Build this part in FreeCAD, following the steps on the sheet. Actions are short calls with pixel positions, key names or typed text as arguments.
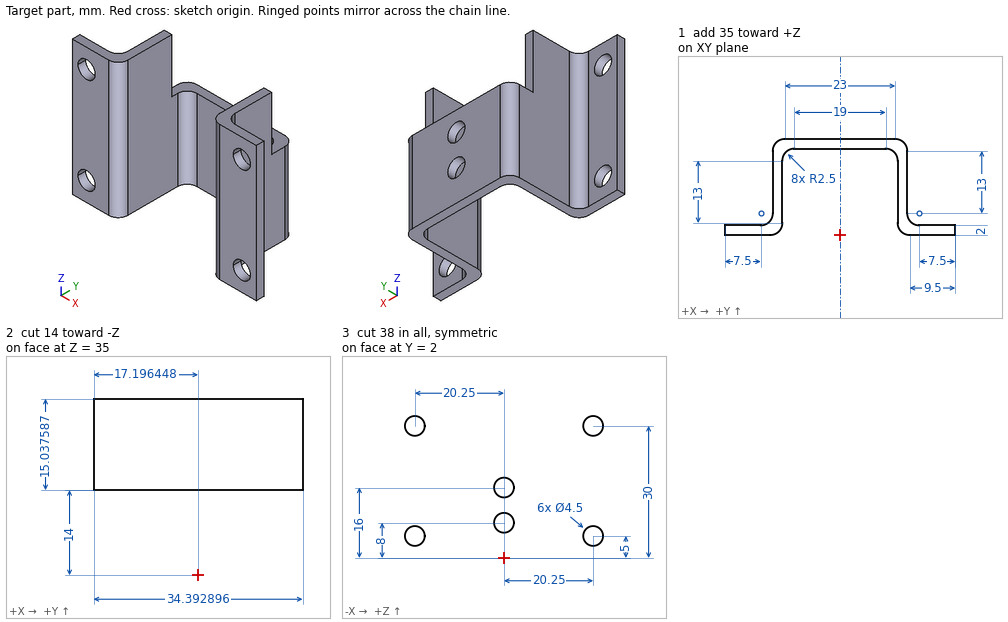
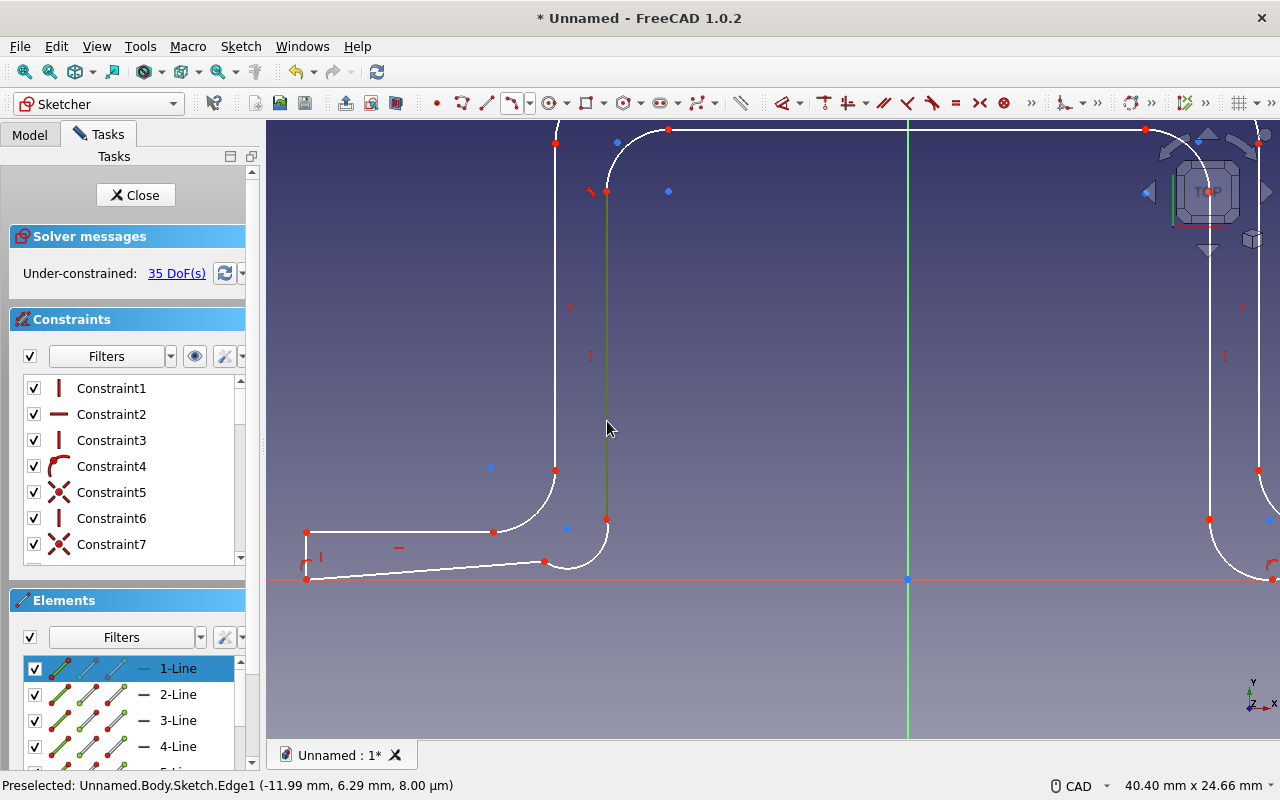
click(572, 568)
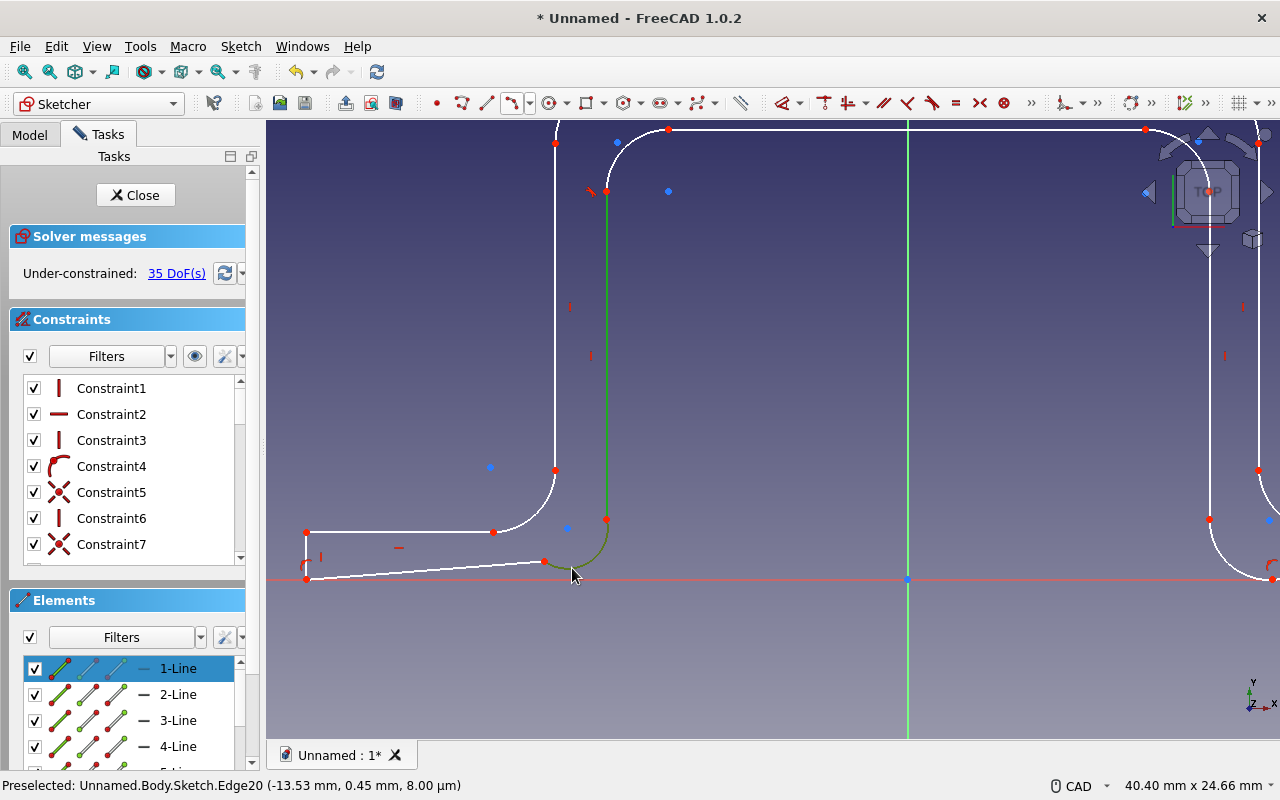
key(t)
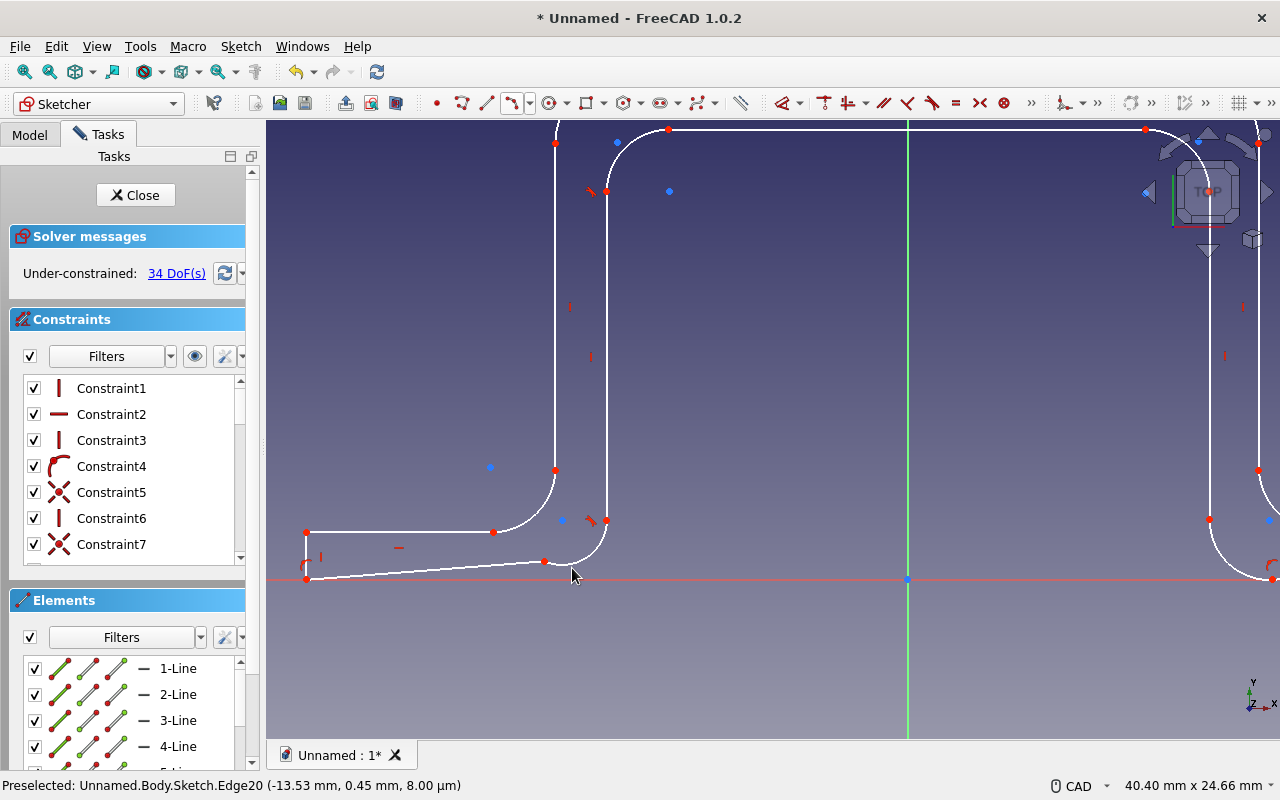
scroll(539, 512, down, 4)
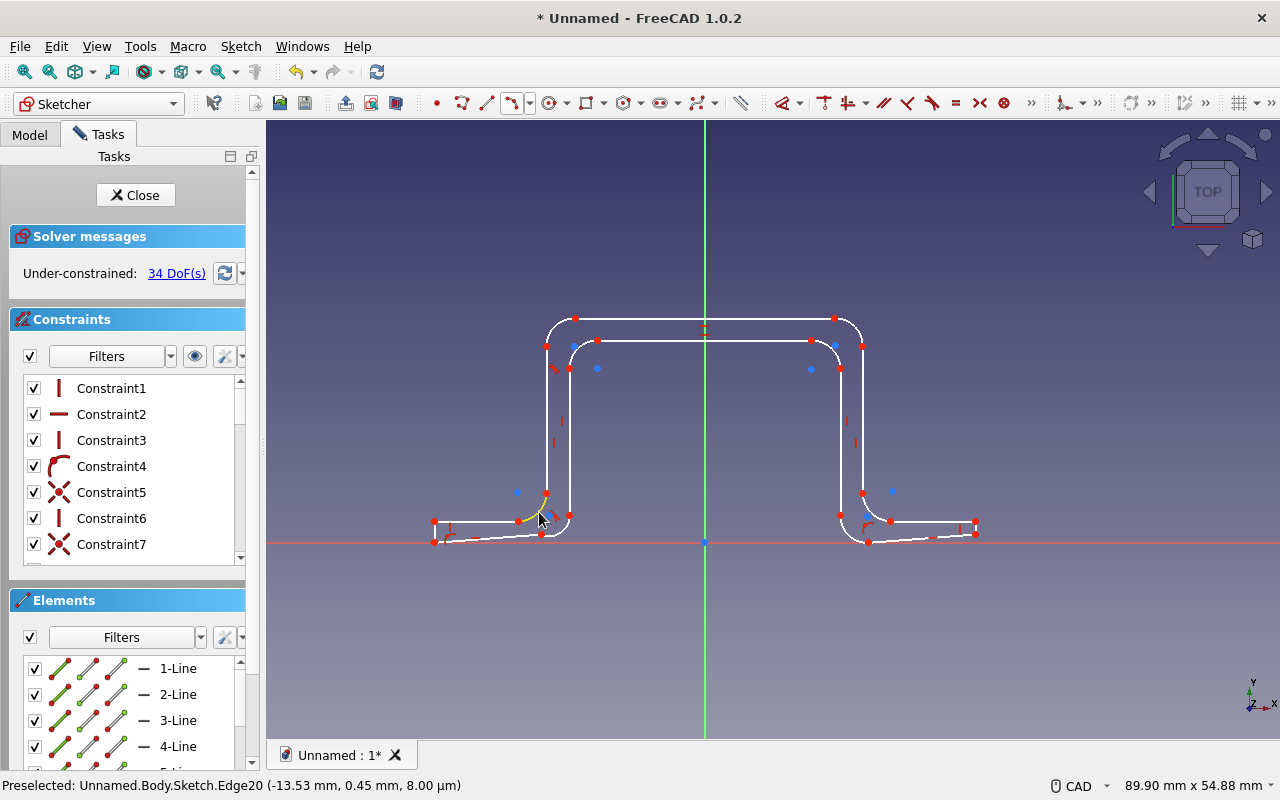
click(662, 341)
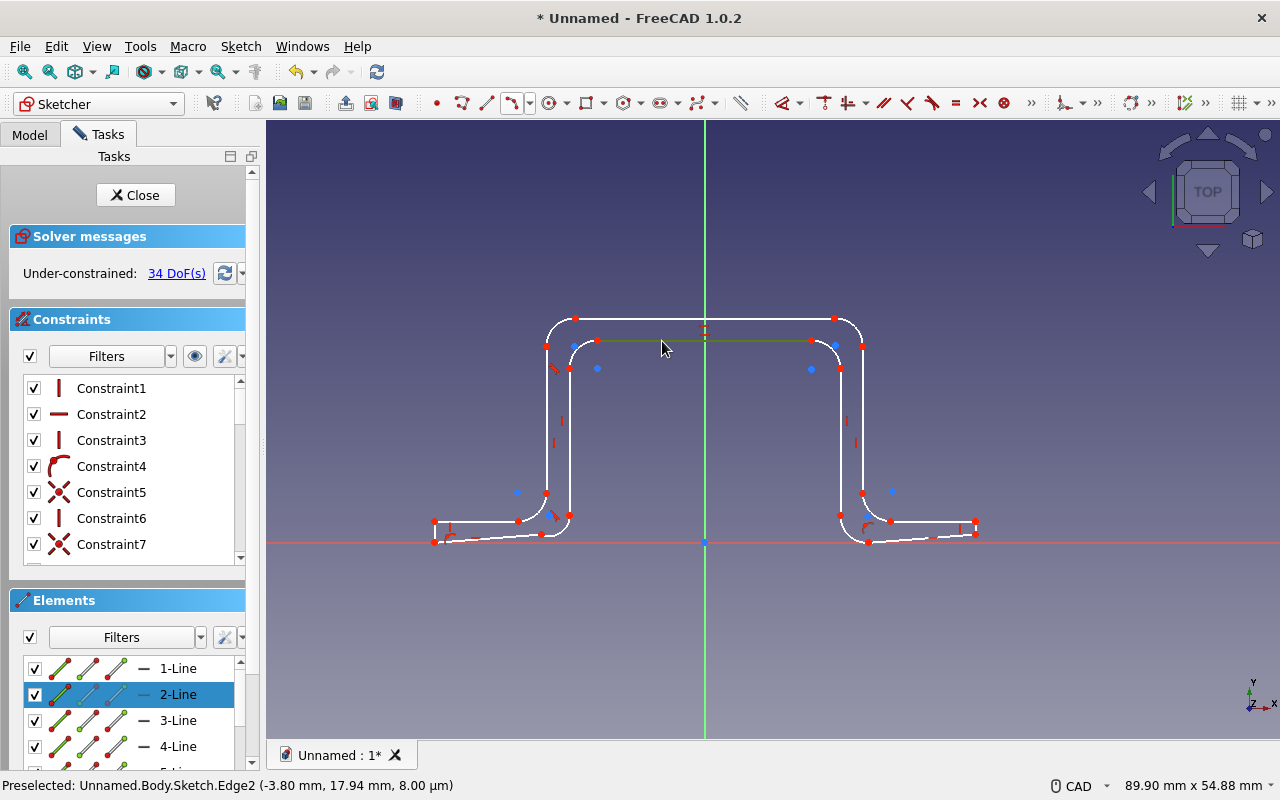
click(585, 344)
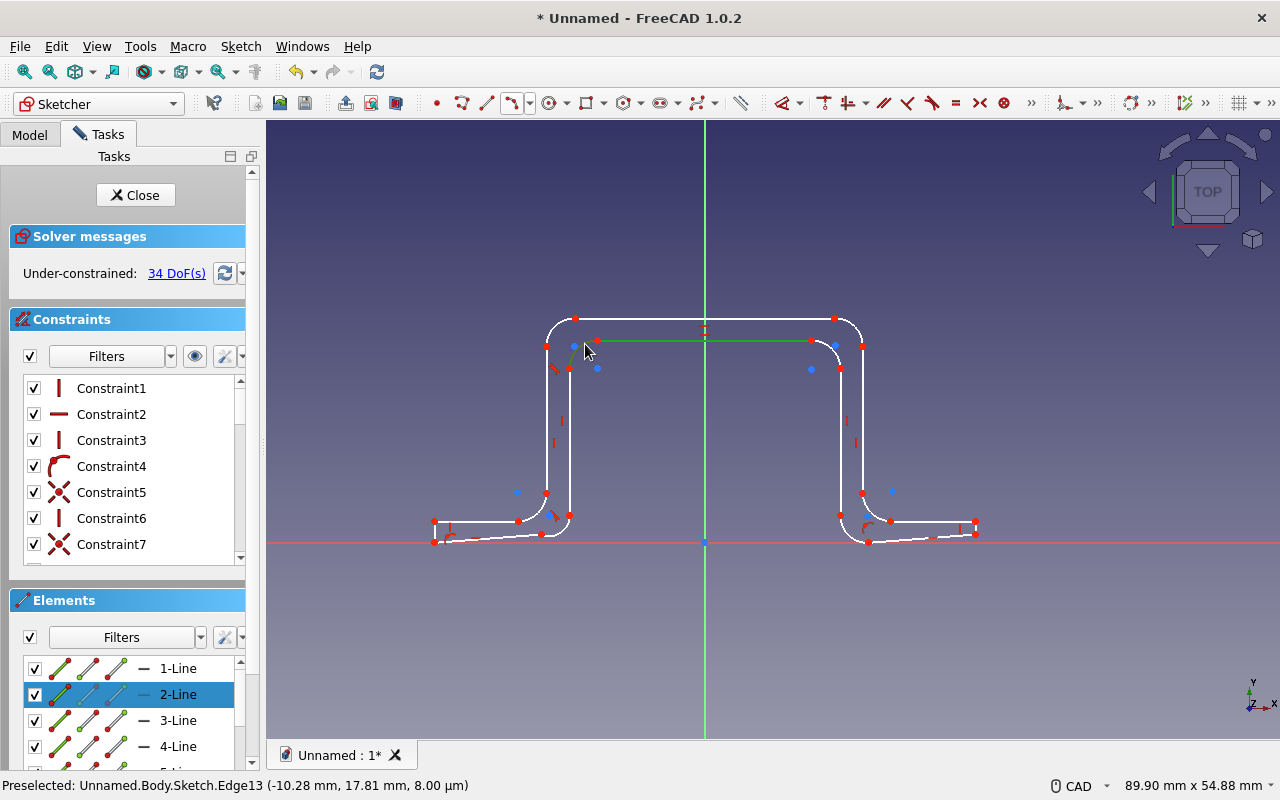
click(932, 104)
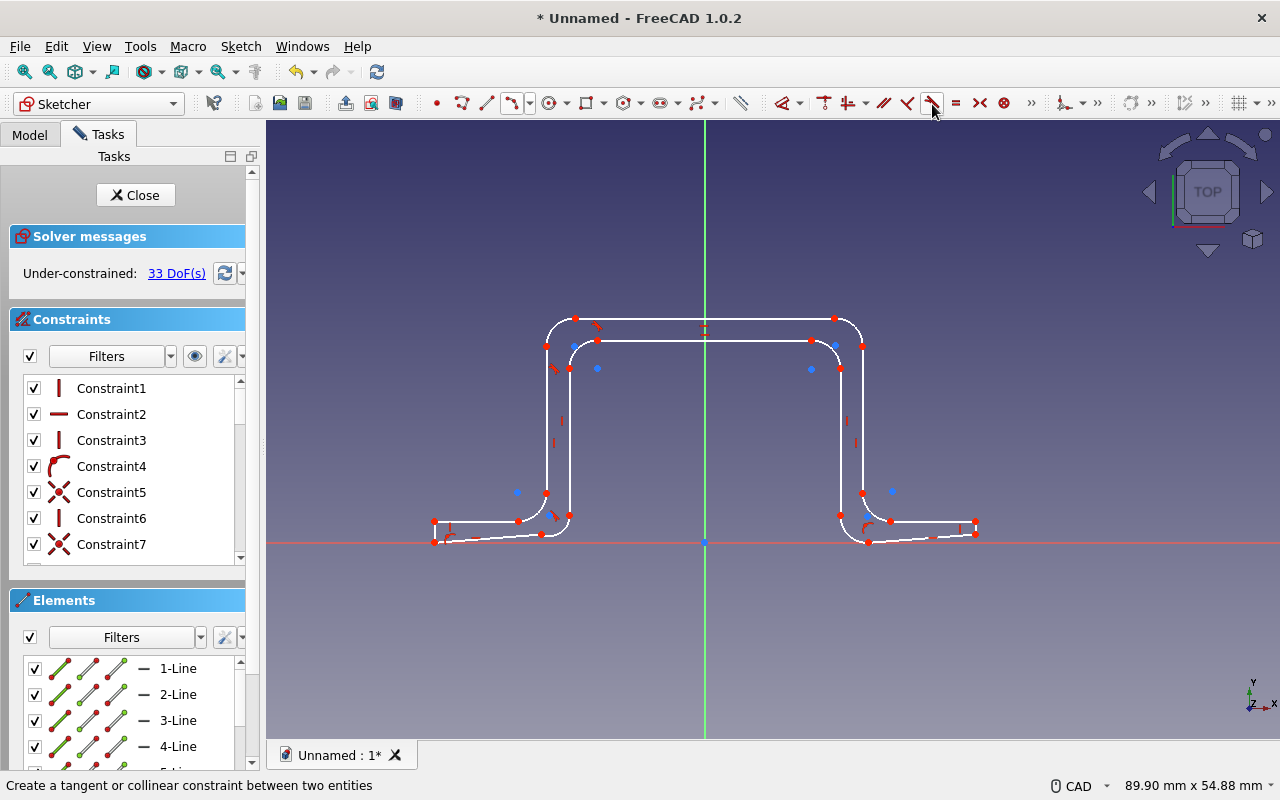
click(662, 341)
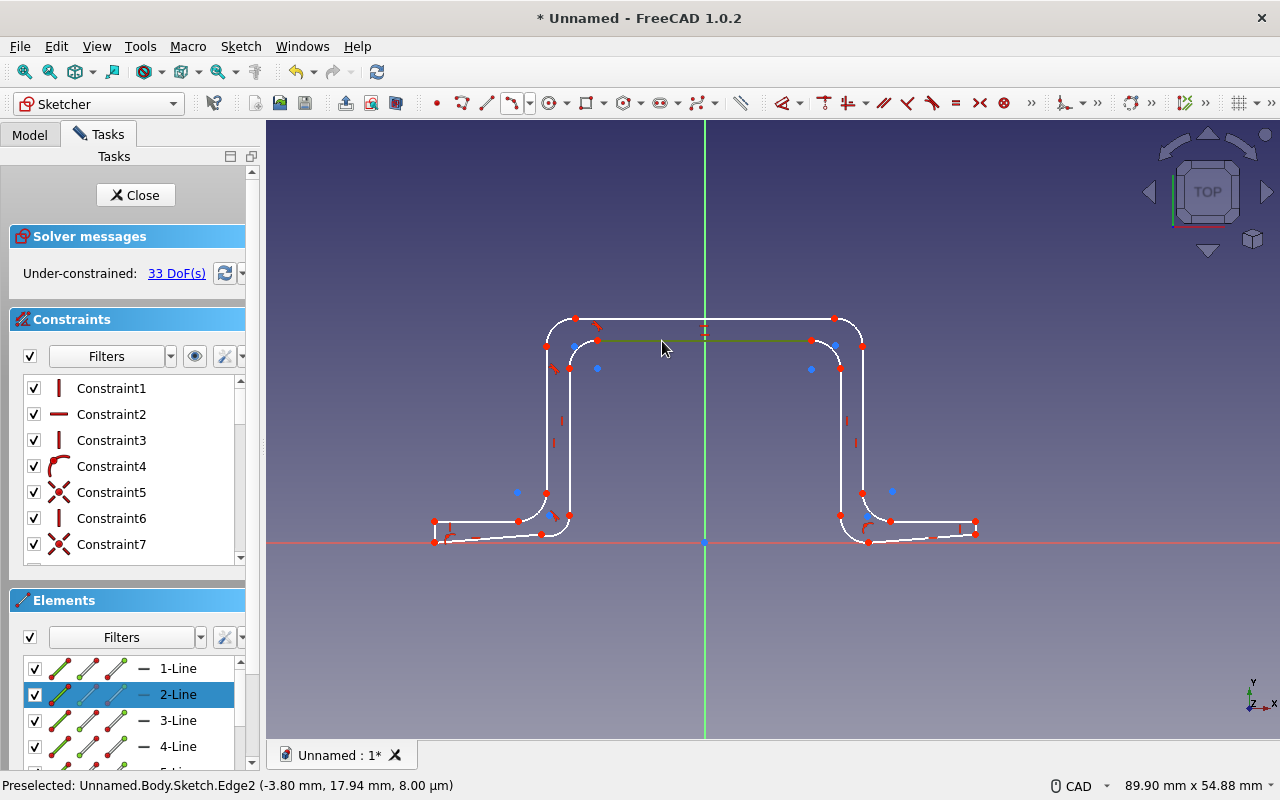
click(837, 356)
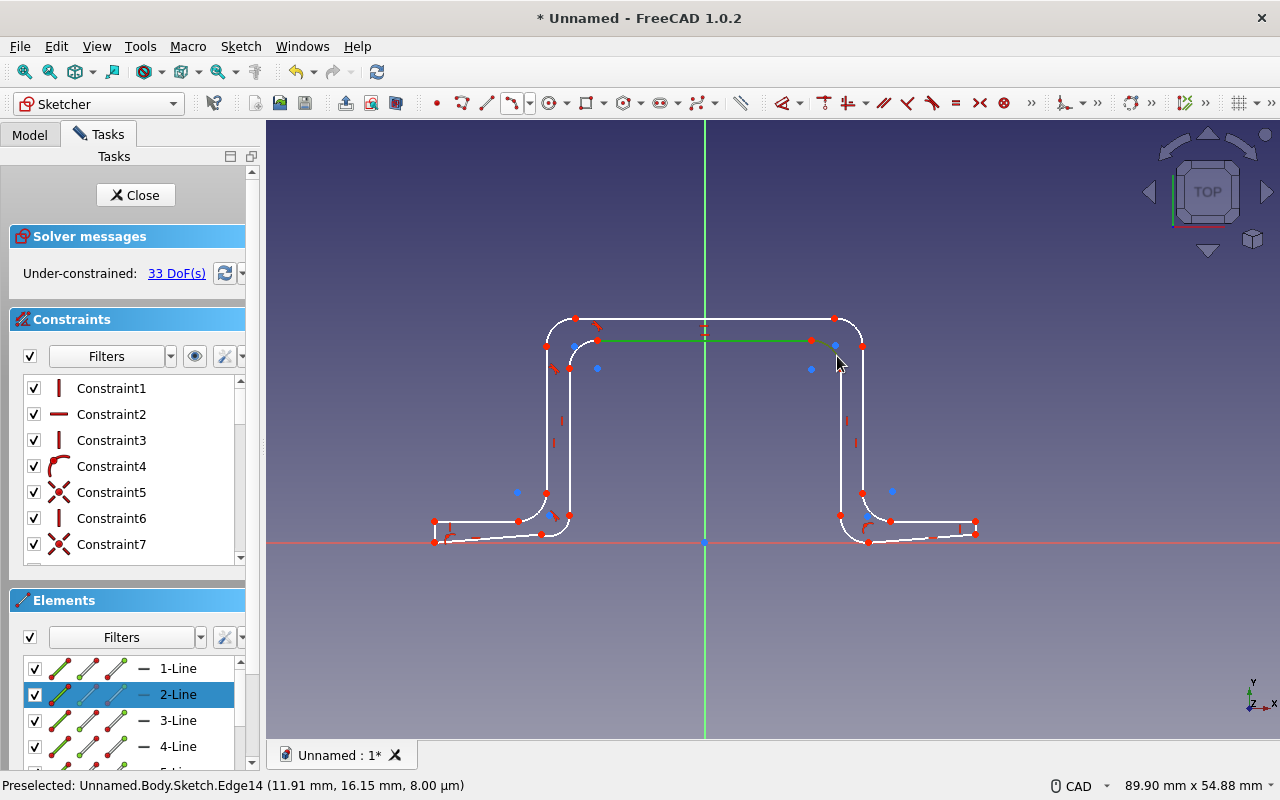
click(932, 104)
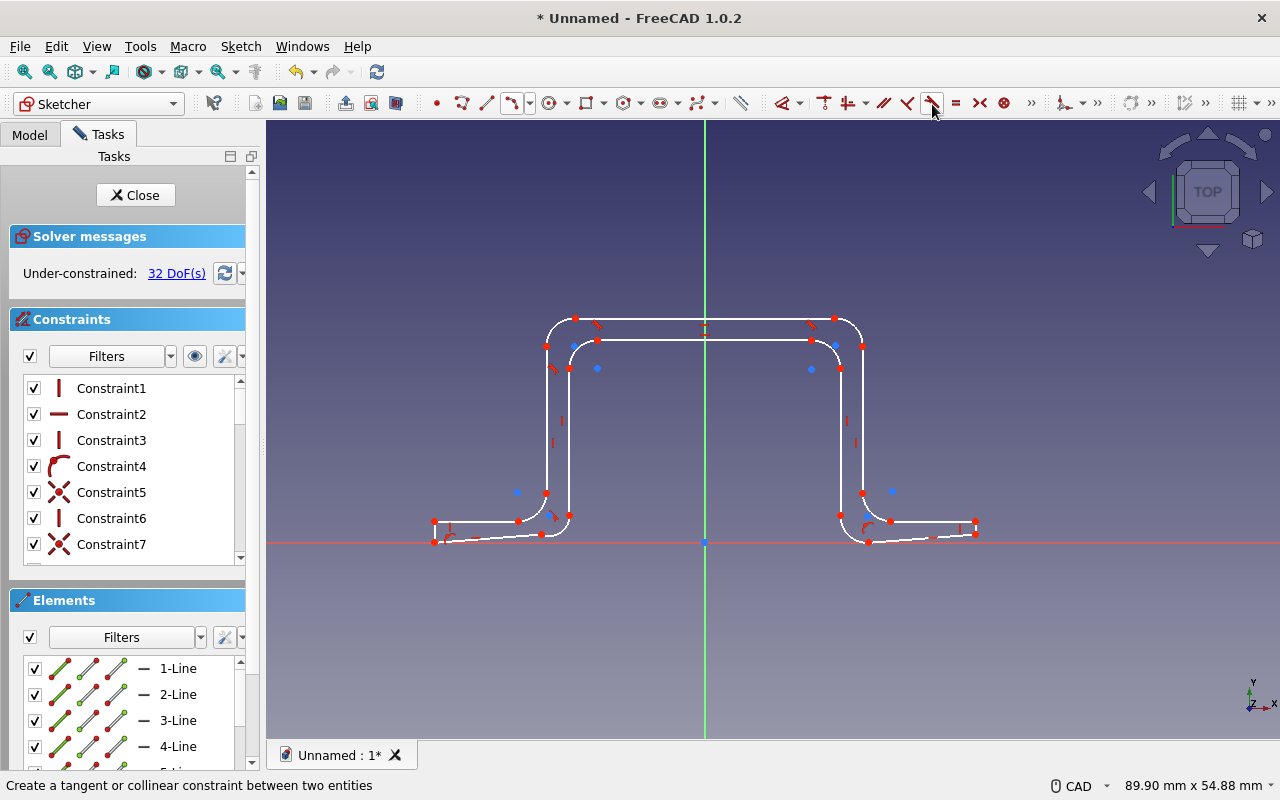
click(841, 413)